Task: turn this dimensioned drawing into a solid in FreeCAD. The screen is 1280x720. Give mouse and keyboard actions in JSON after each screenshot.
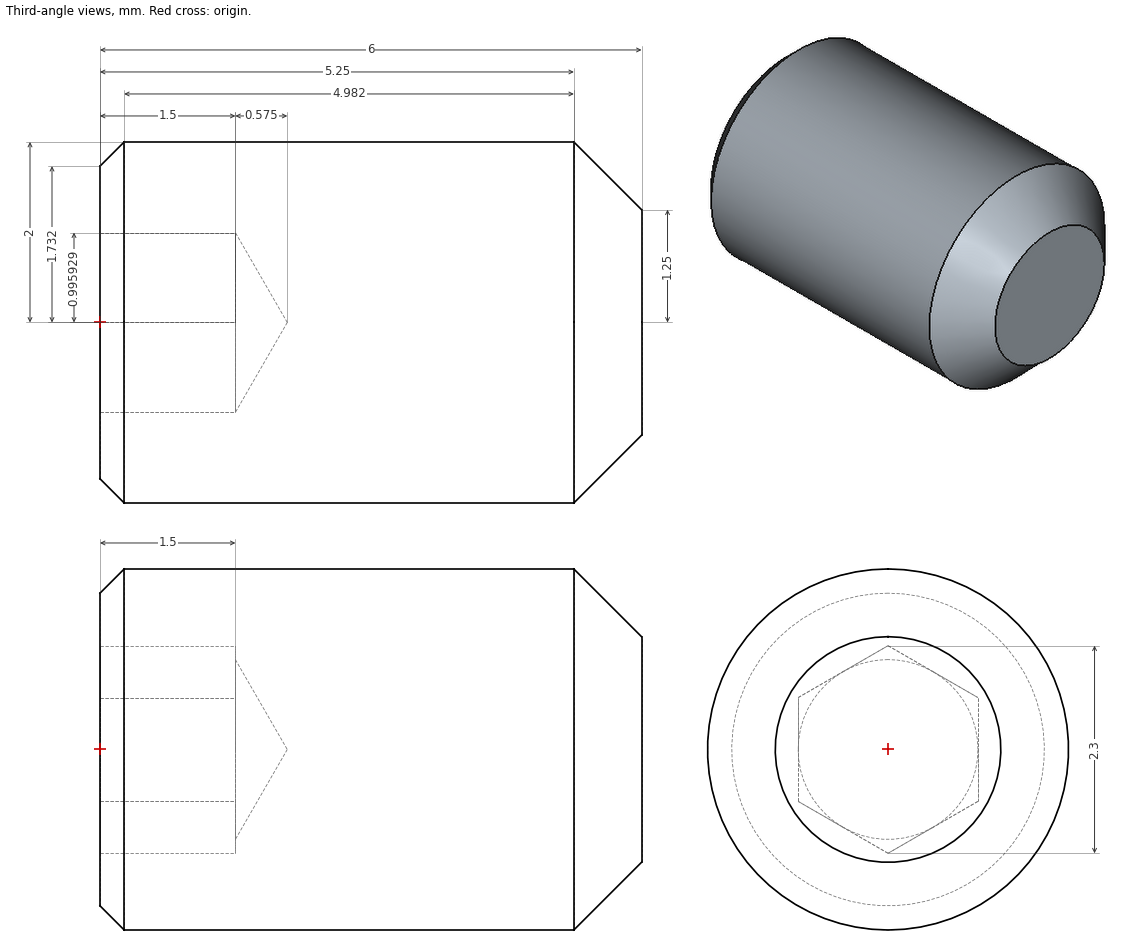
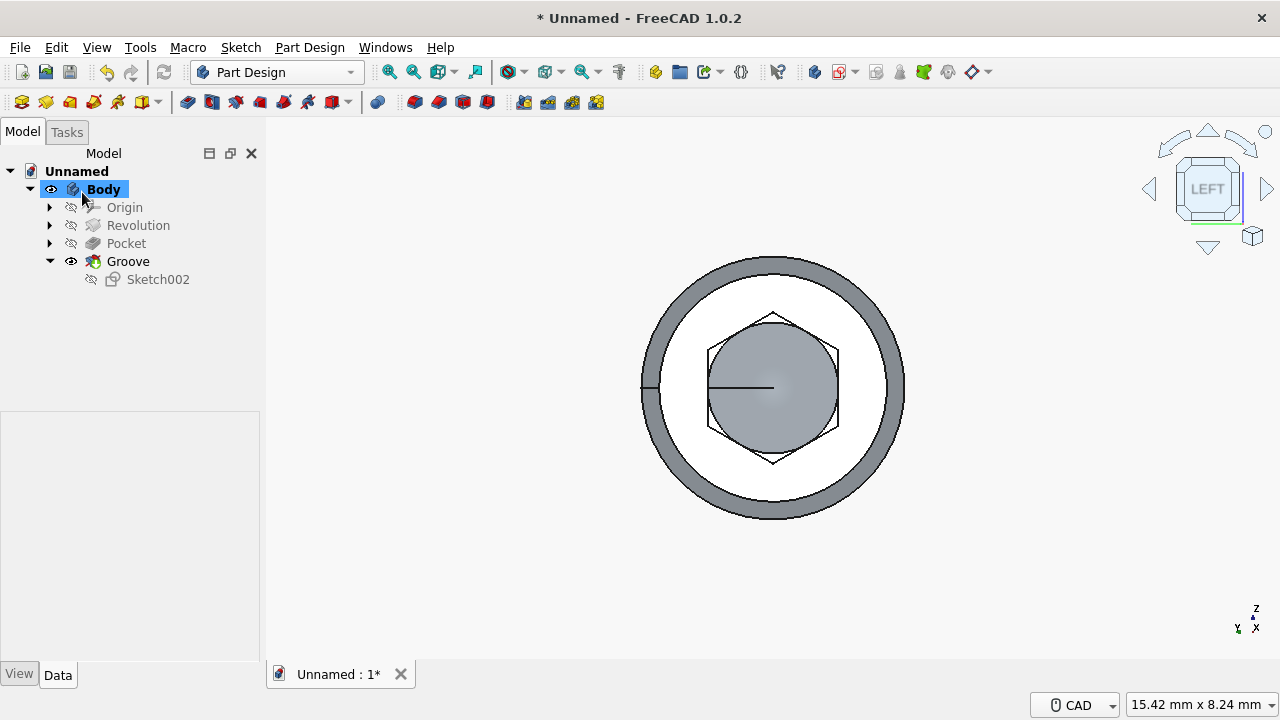
{"action": "key", "text": "0"}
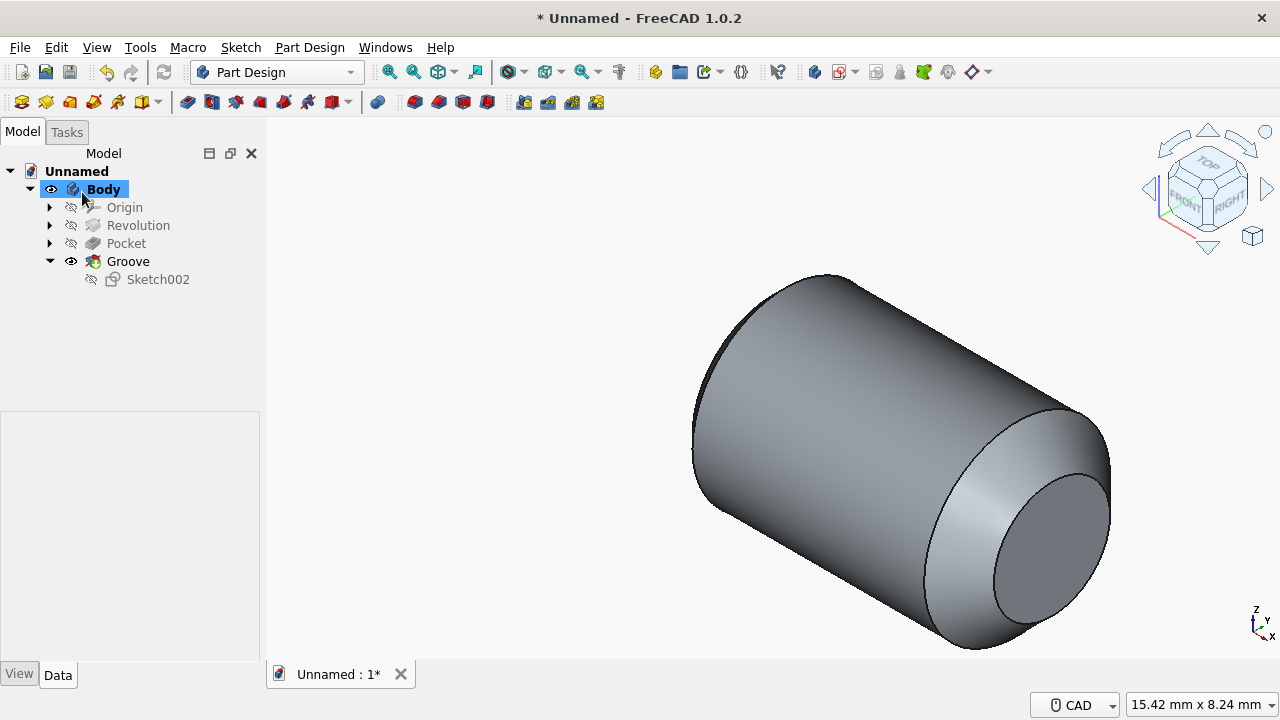
{"action": "left_click", "coordinate": [390, 72]}